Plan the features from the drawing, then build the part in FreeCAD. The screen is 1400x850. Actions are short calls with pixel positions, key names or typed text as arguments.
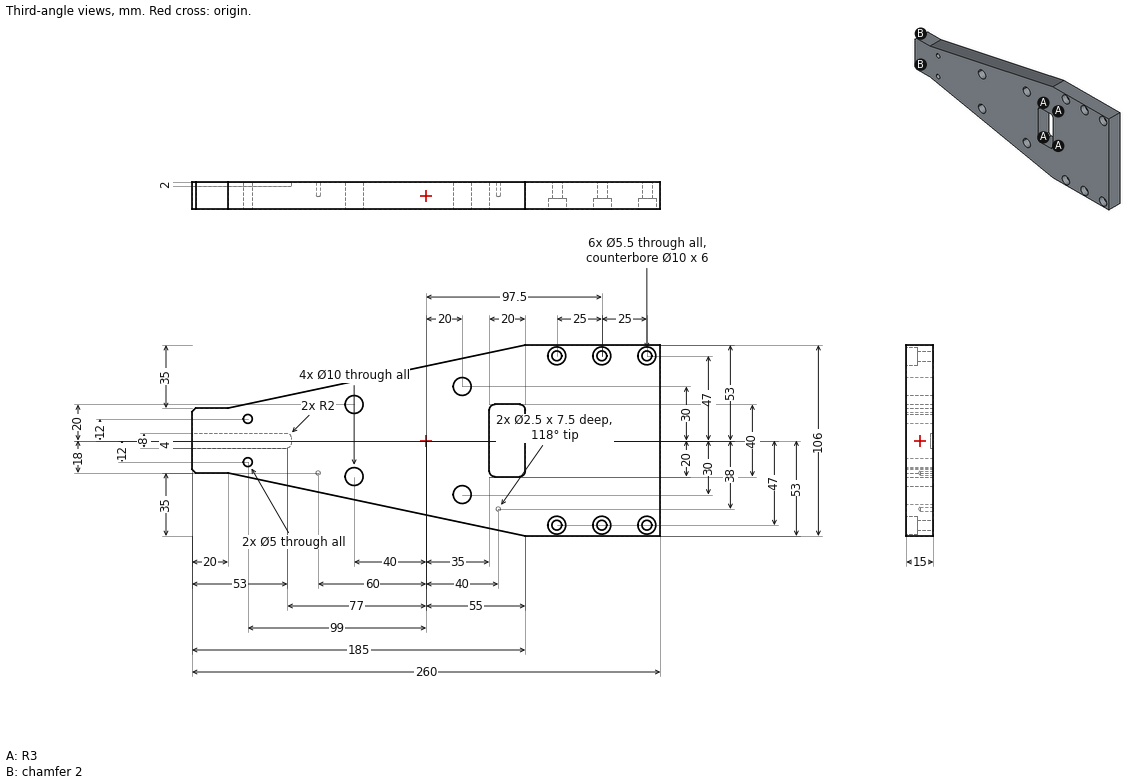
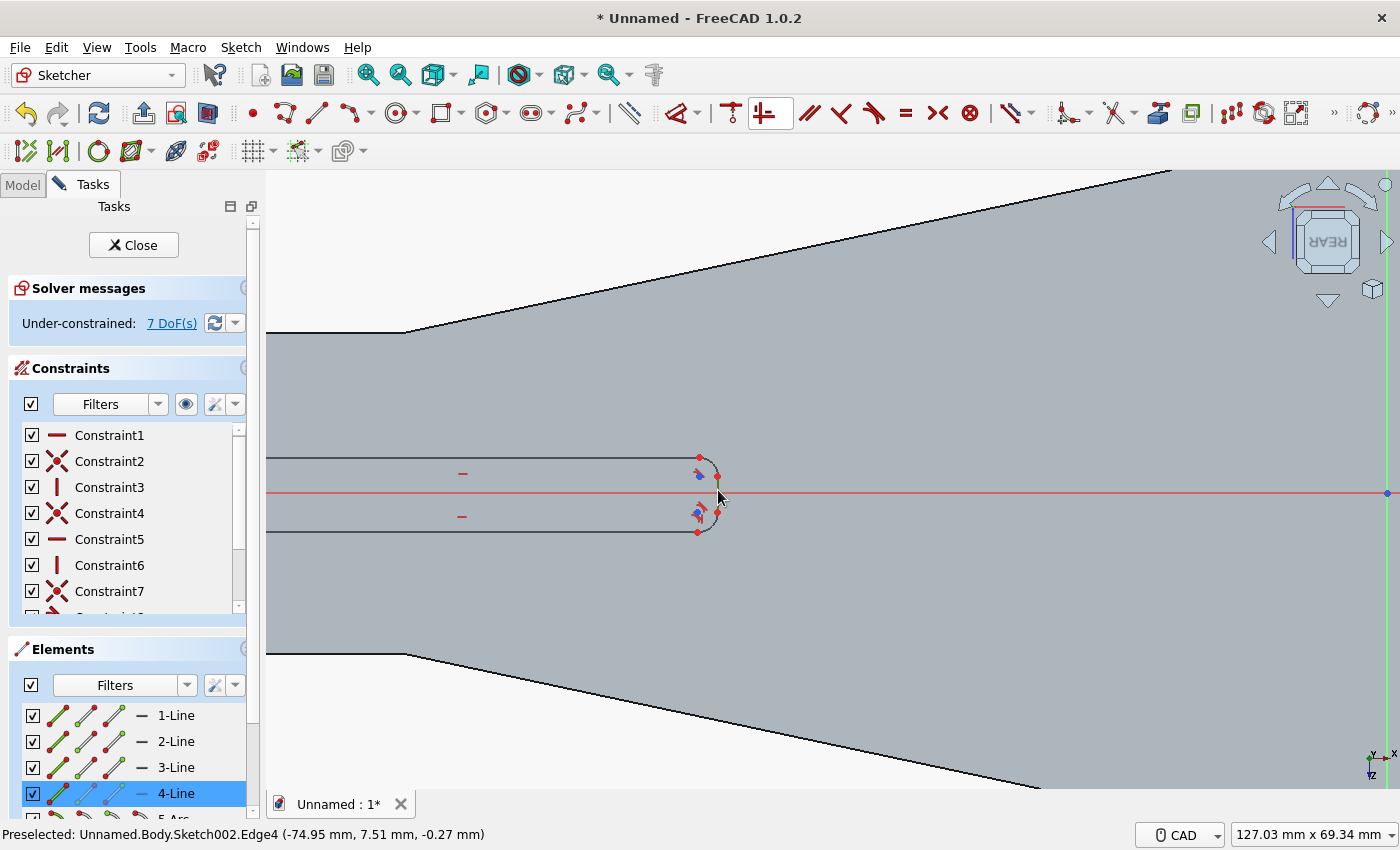
click(712, 463)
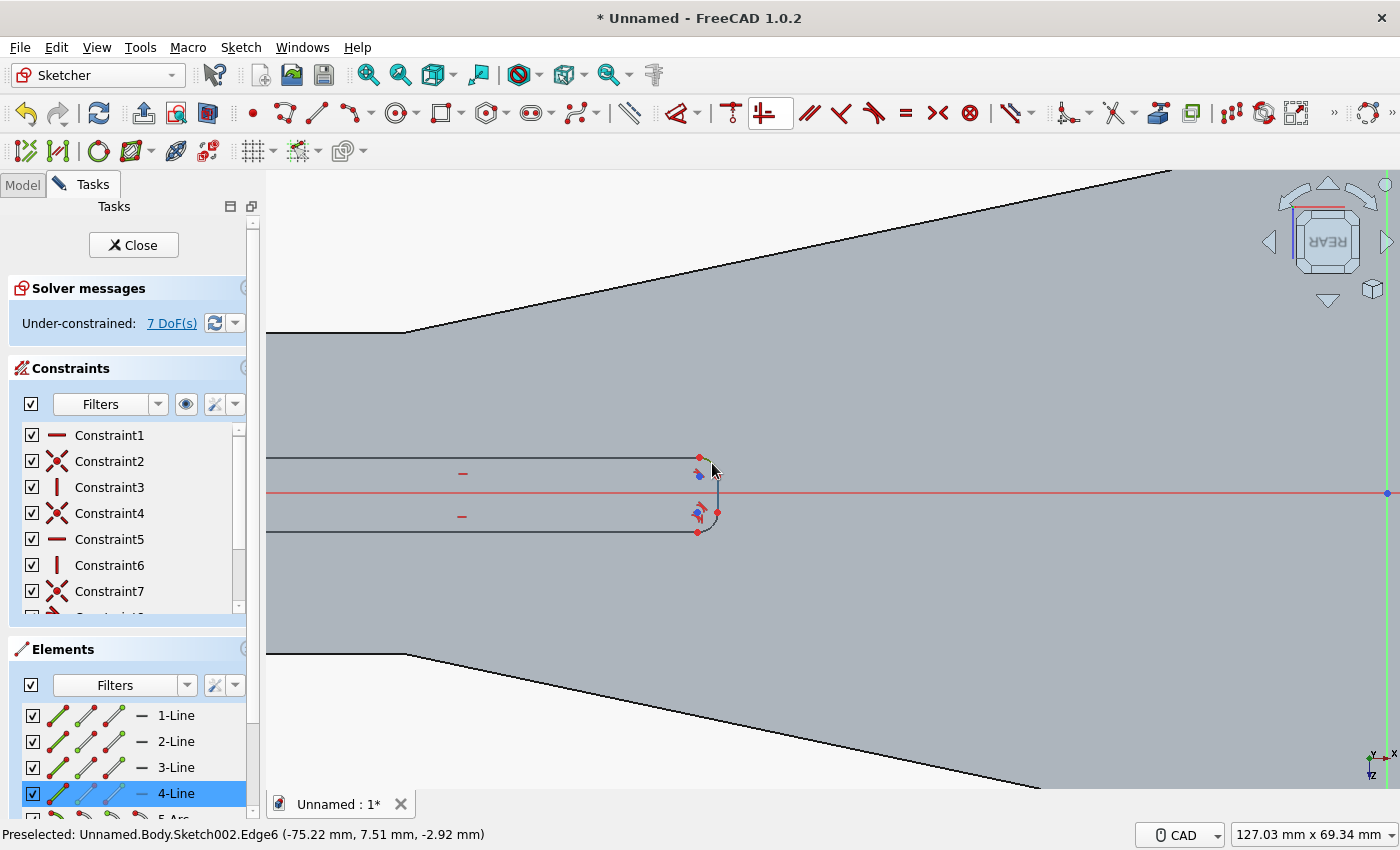
click(874, 114)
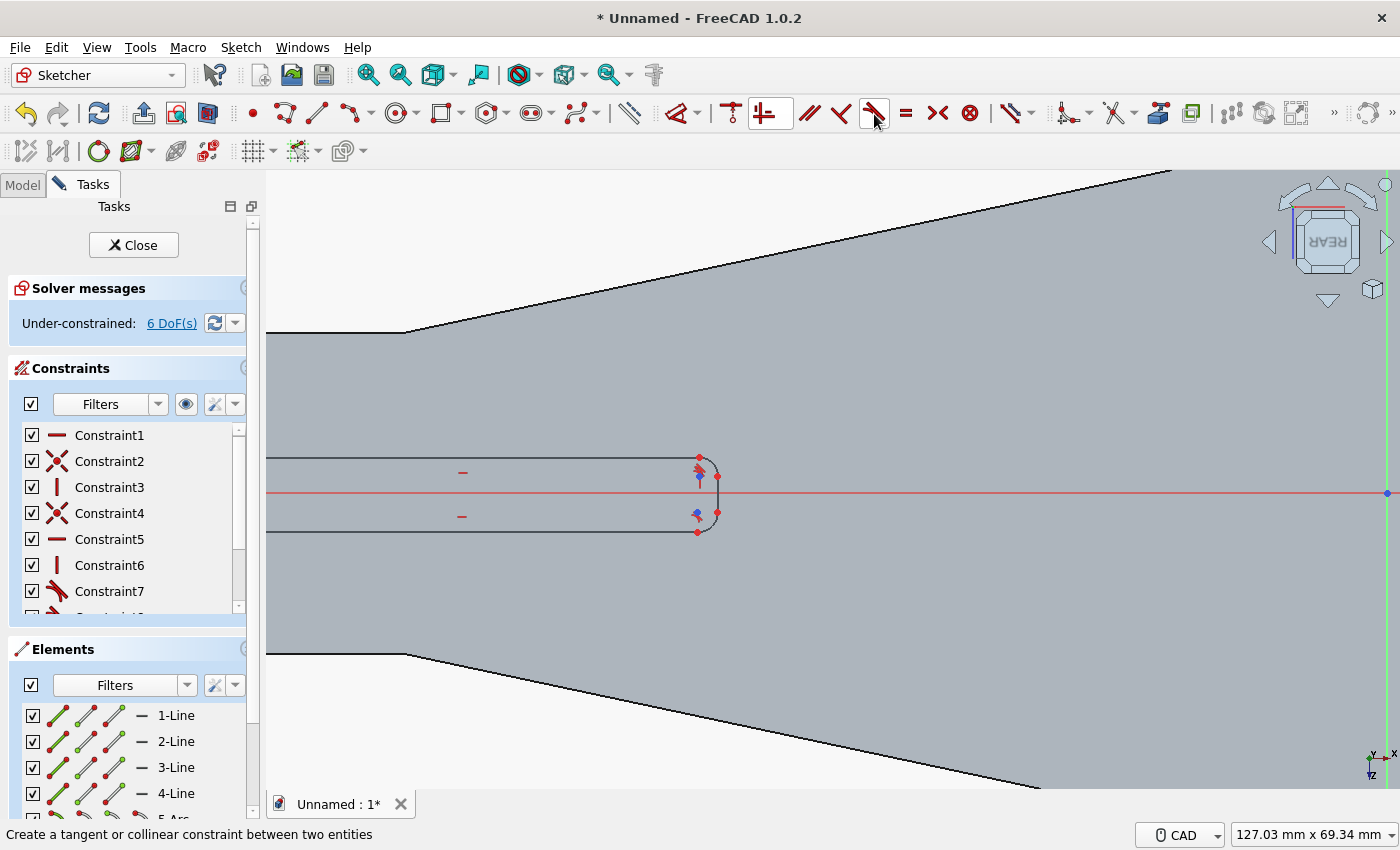
scroll(707, 530, up, 2)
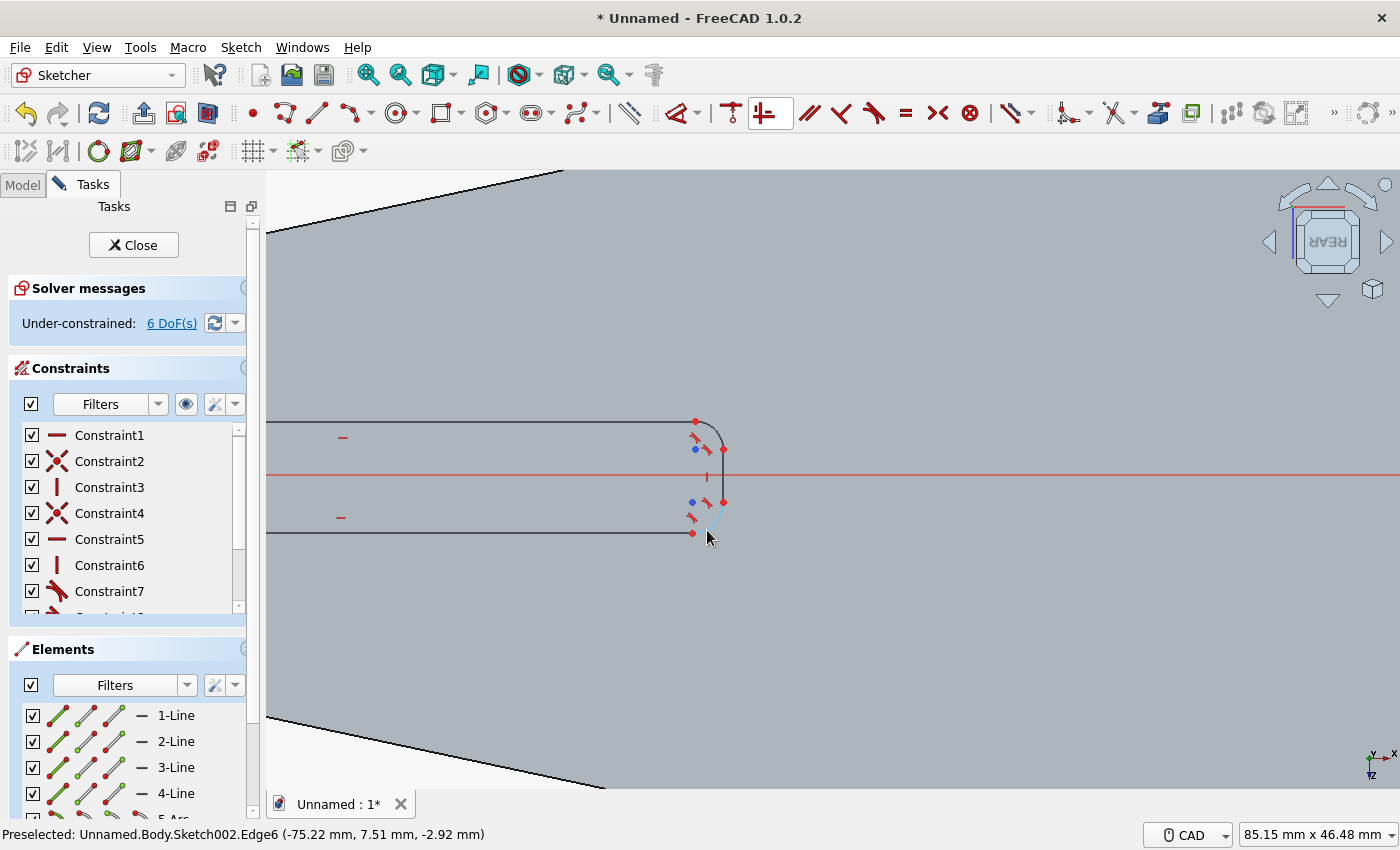
click(707, 530)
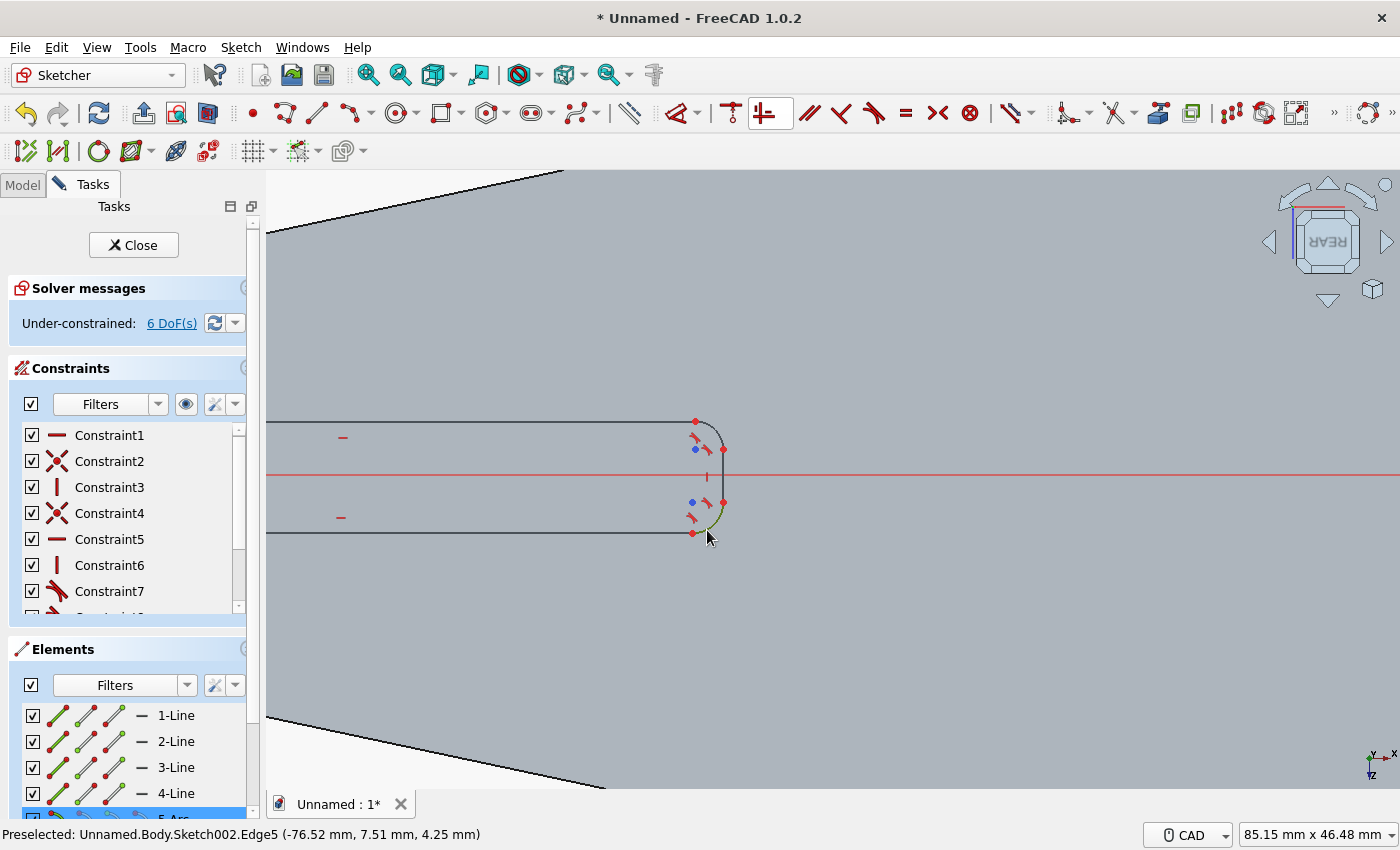
click(720, 437)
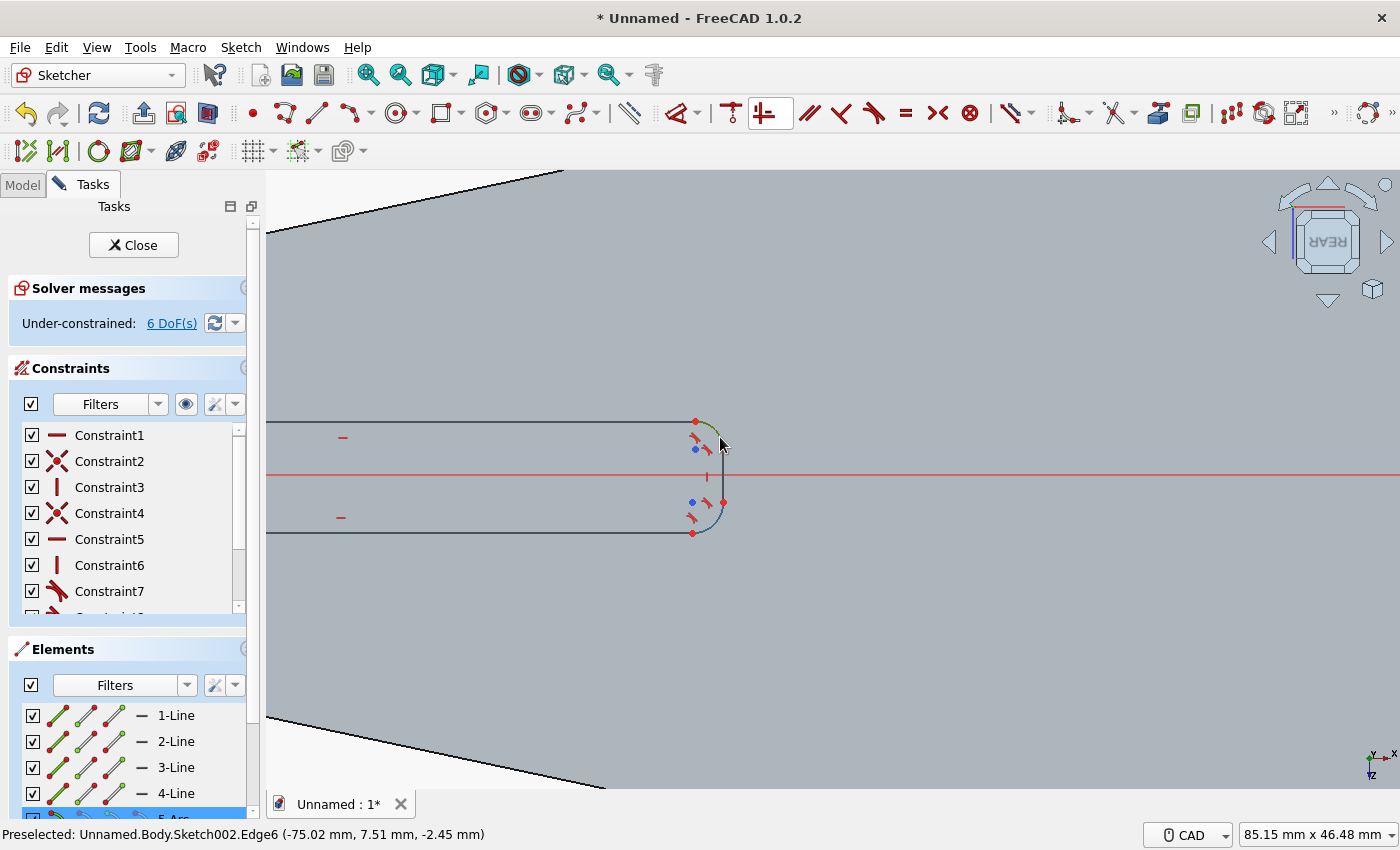
click(906, 114)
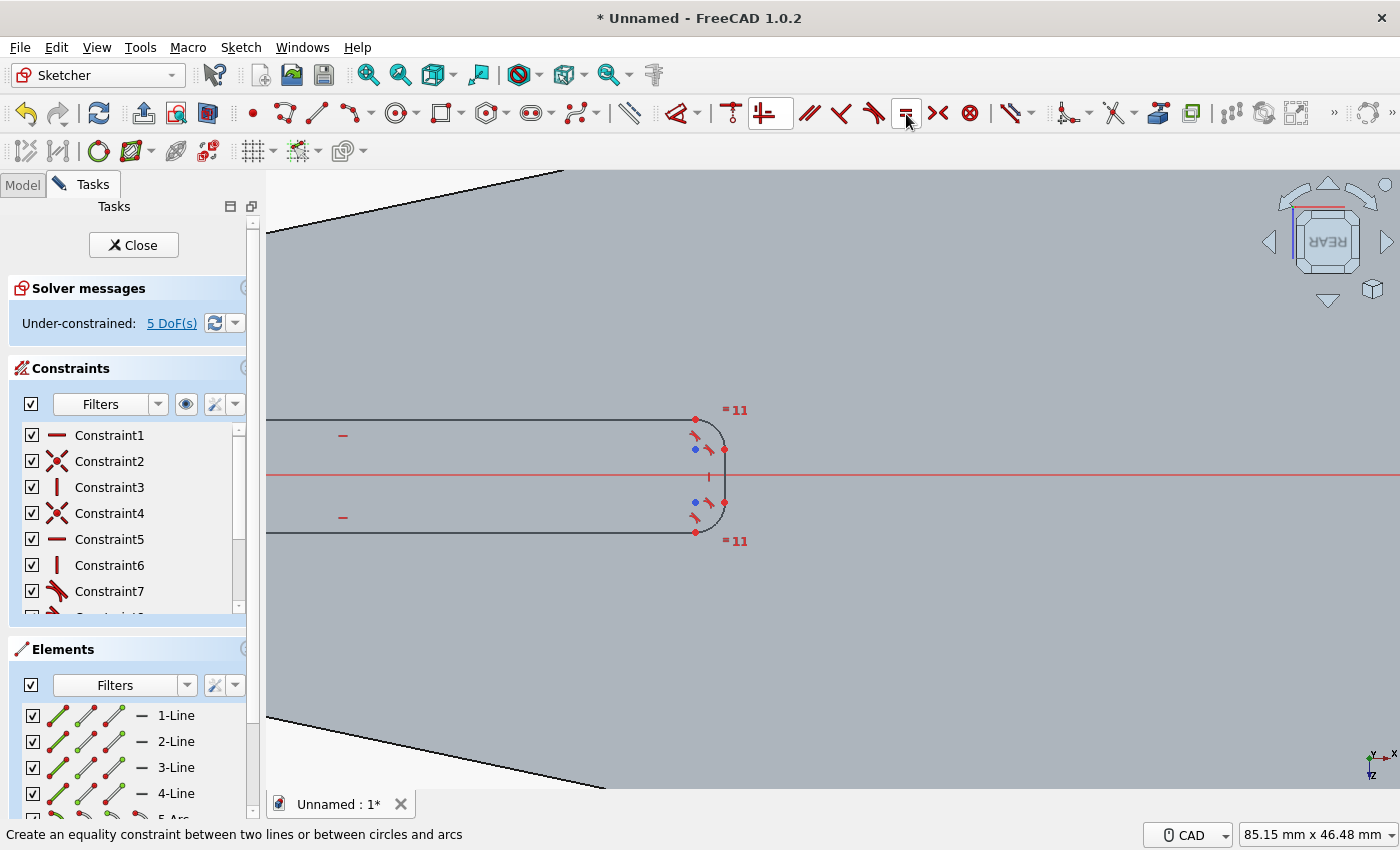
key(d)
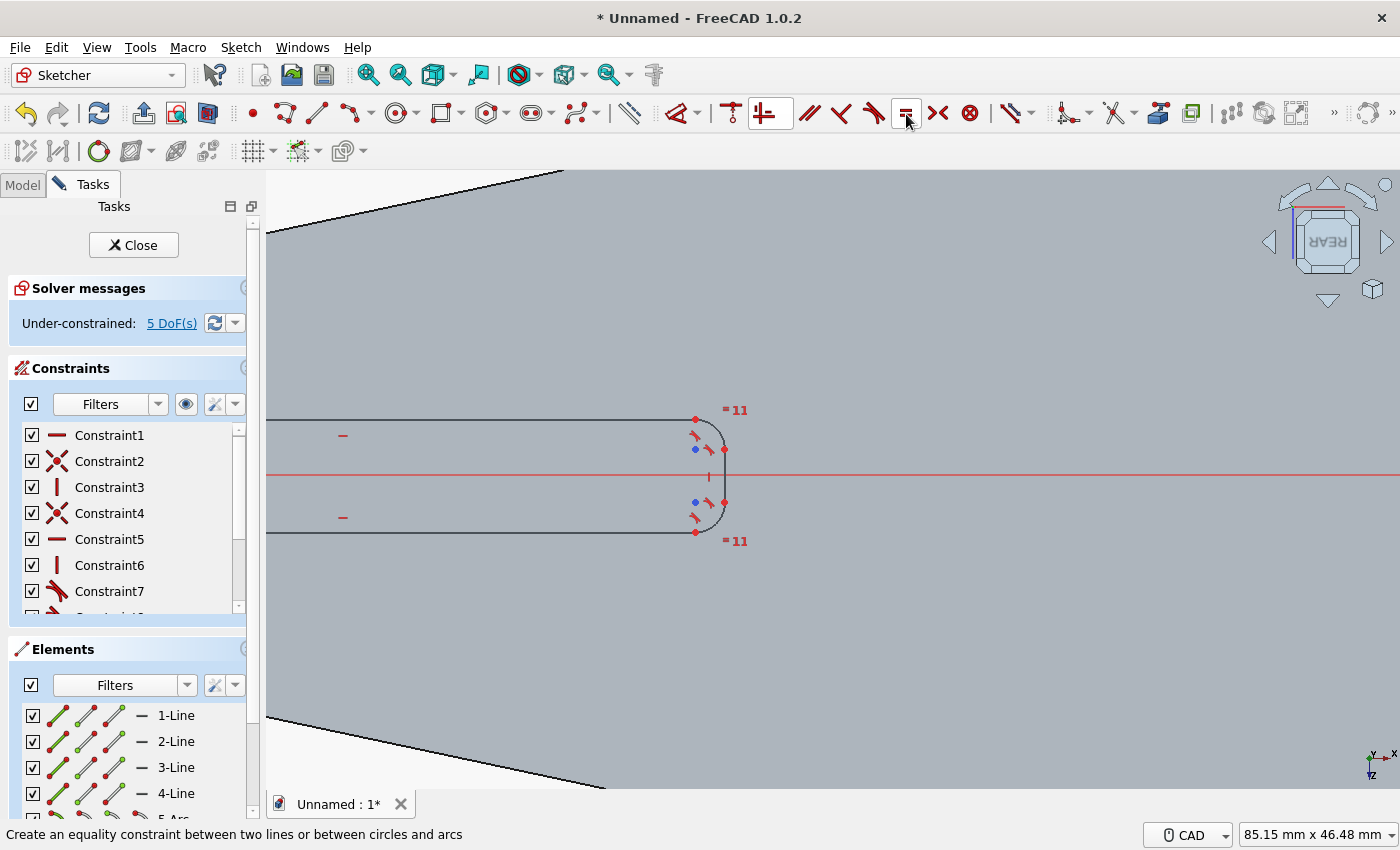
scroll(709, 529, up, 2)